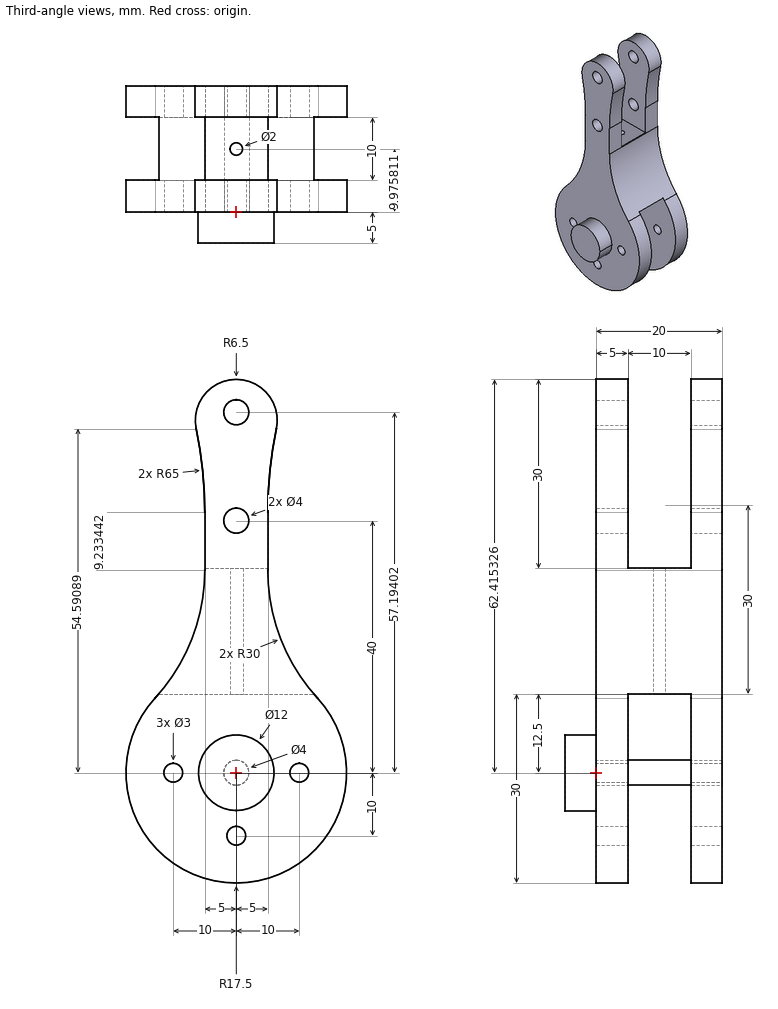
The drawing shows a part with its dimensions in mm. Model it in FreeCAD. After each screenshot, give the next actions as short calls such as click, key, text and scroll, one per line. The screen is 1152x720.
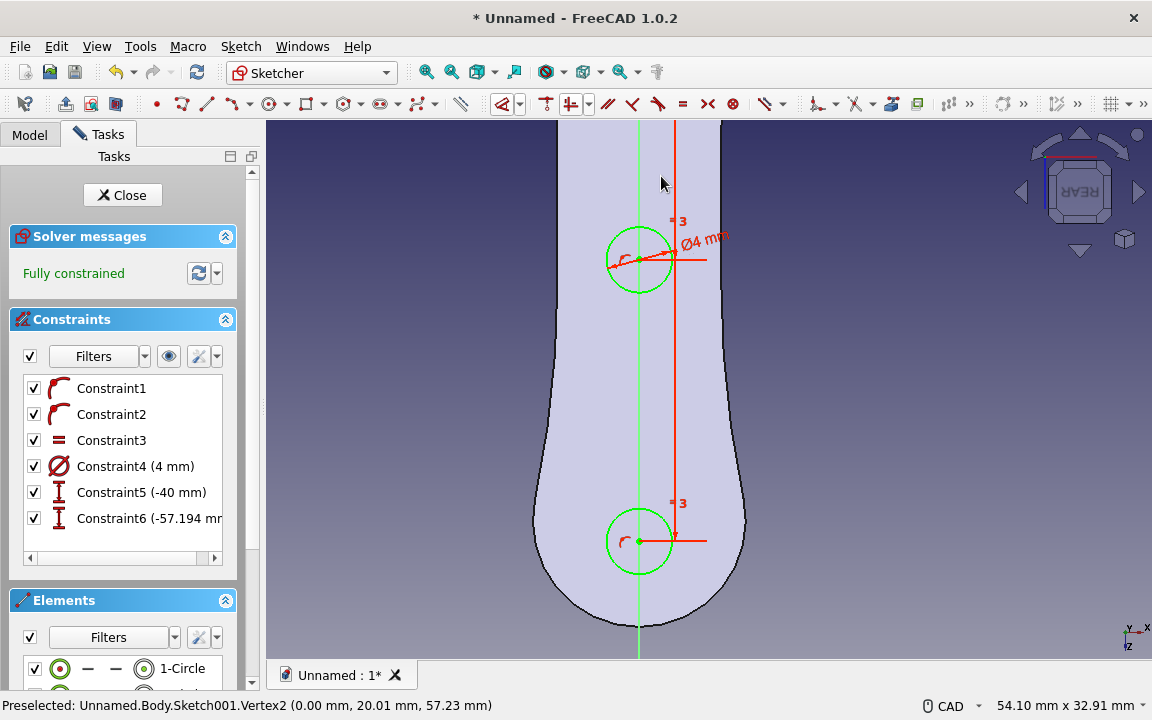
click(123, 195)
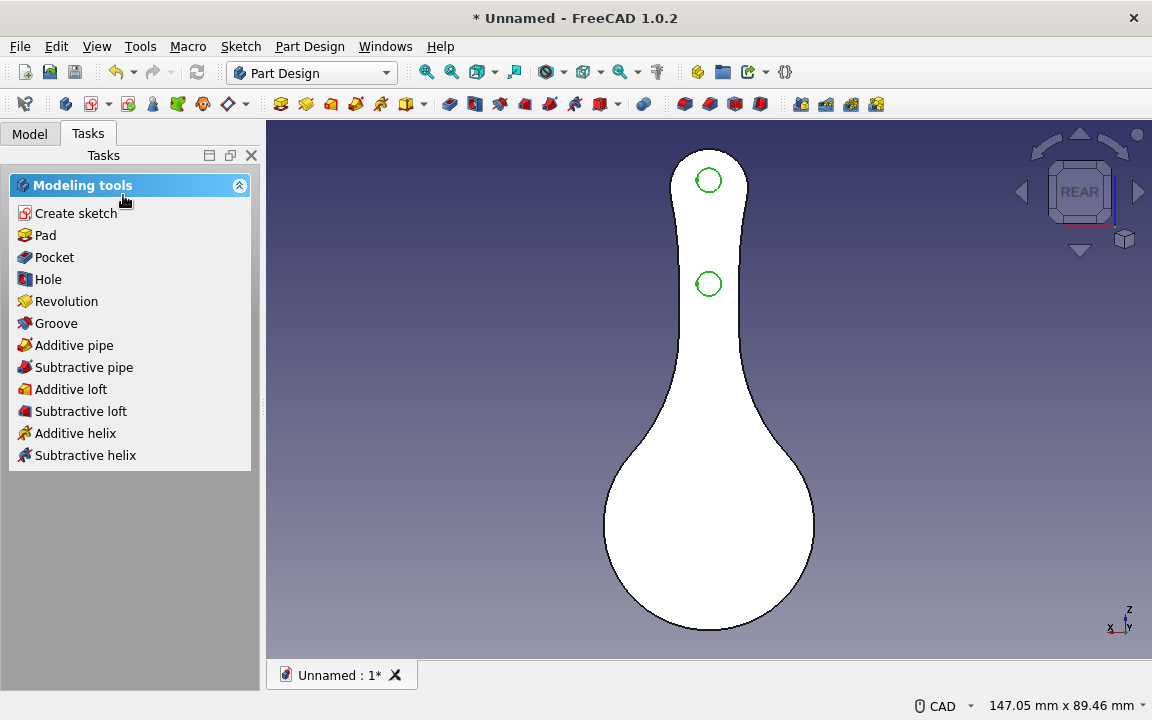
click(450, 104)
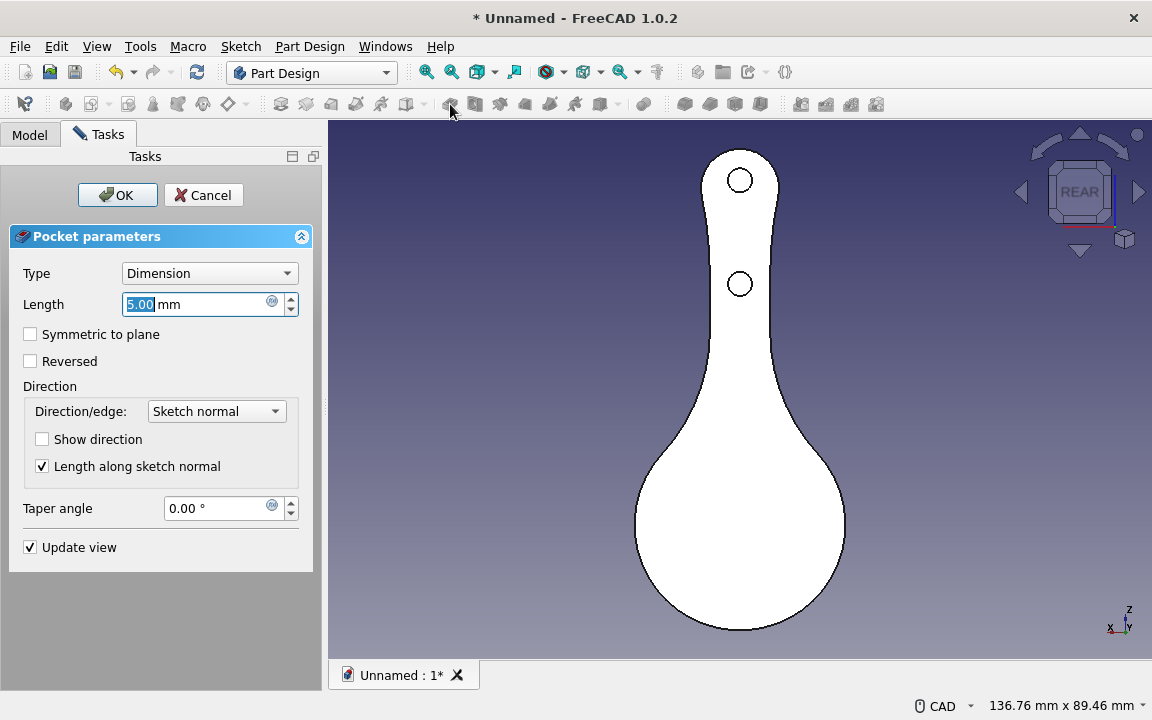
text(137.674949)
key(Tab)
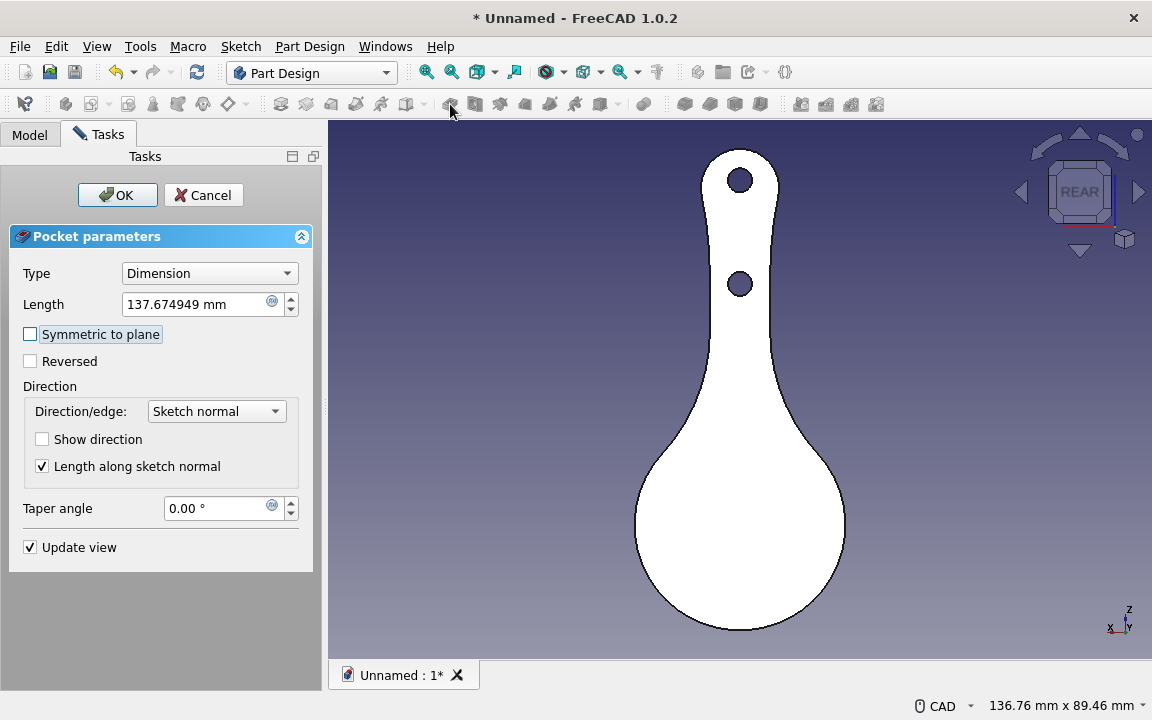
click(31, 334)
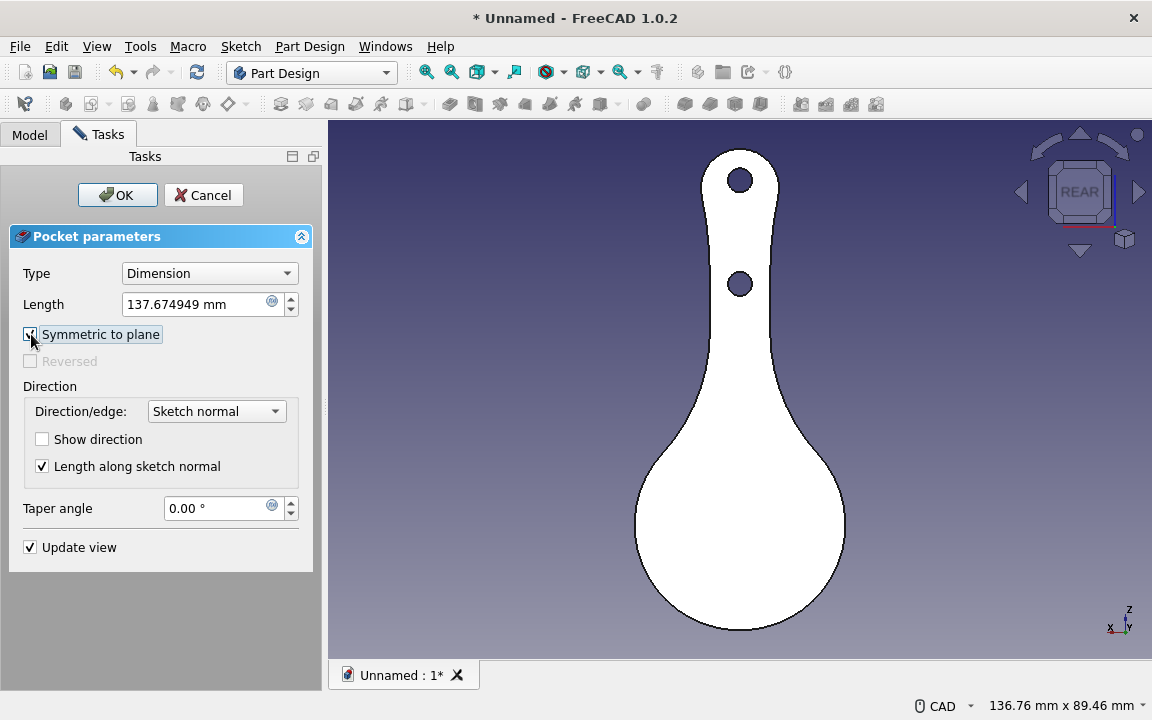
click(118, 195)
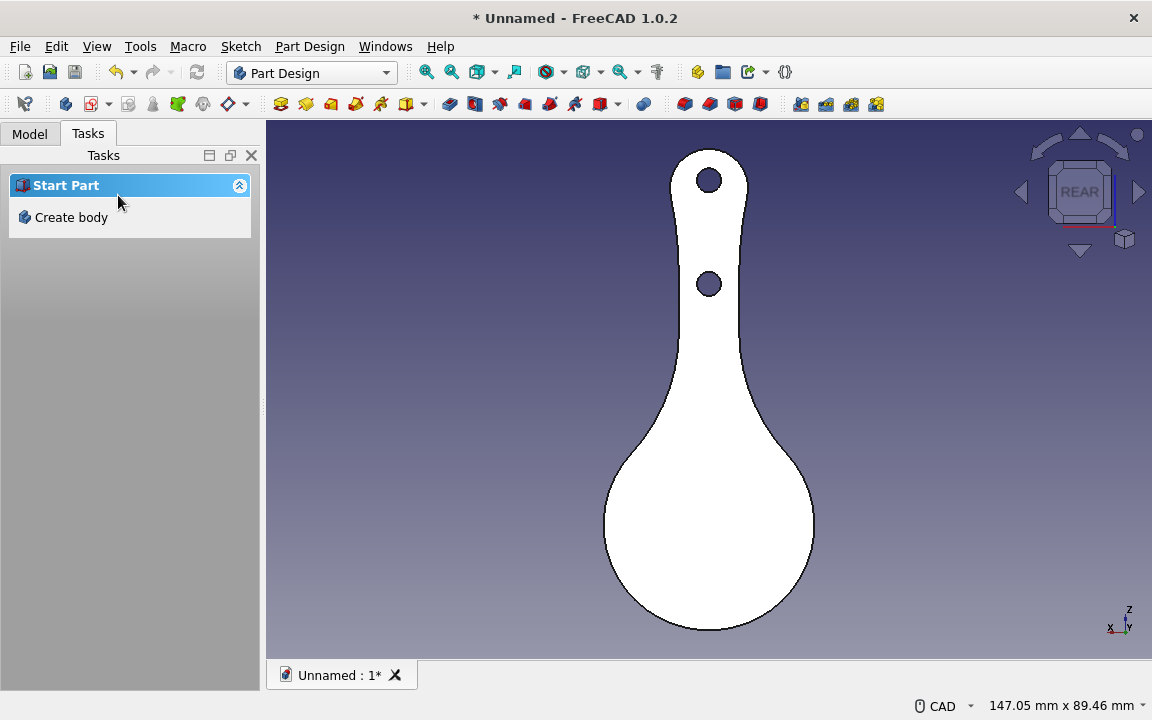
click(709, 526)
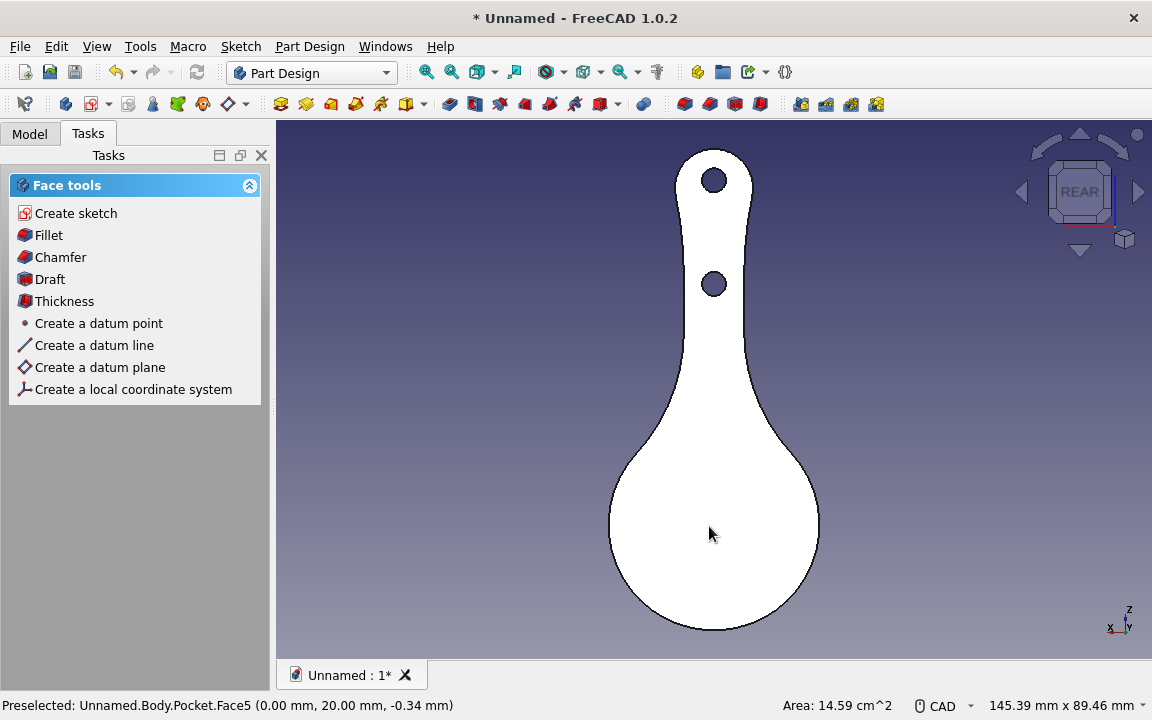
click(90, 104)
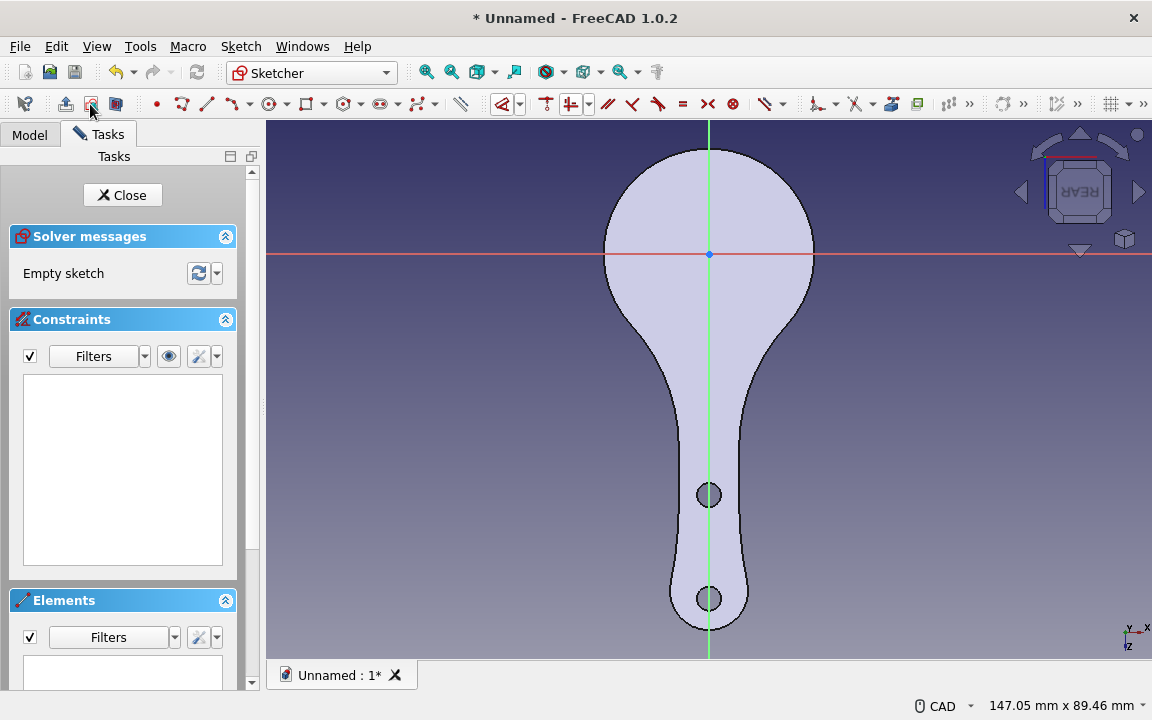
scroll(714, 243, up, 13)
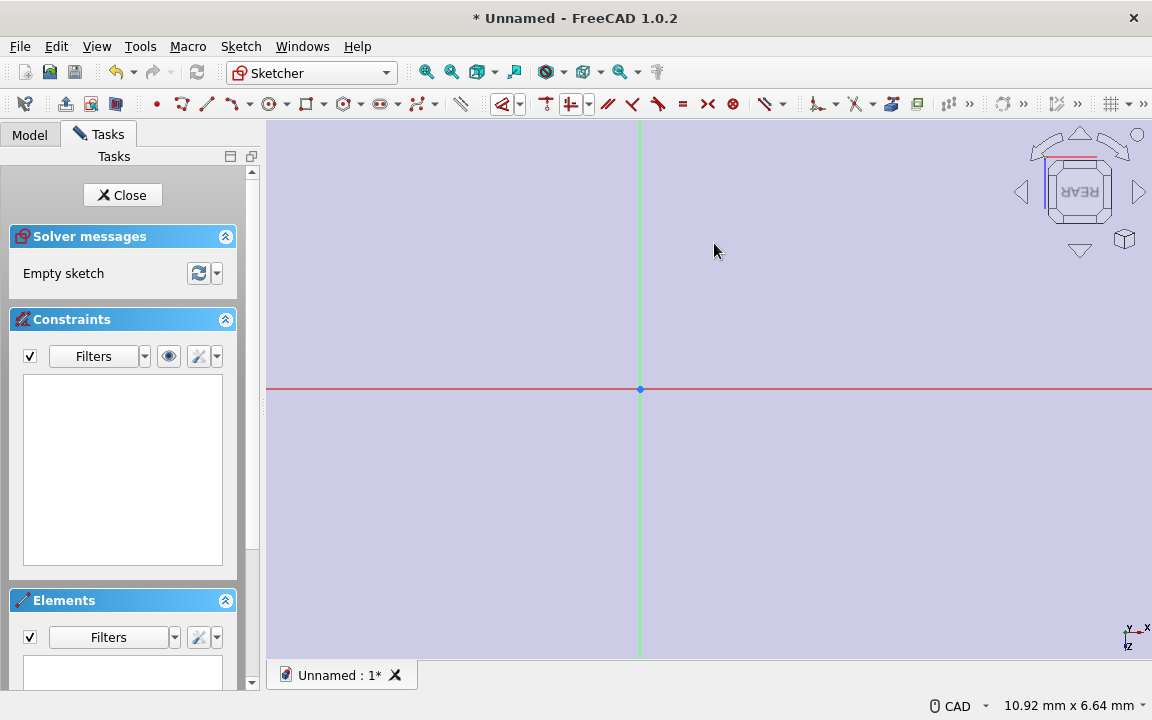
click(268, 104)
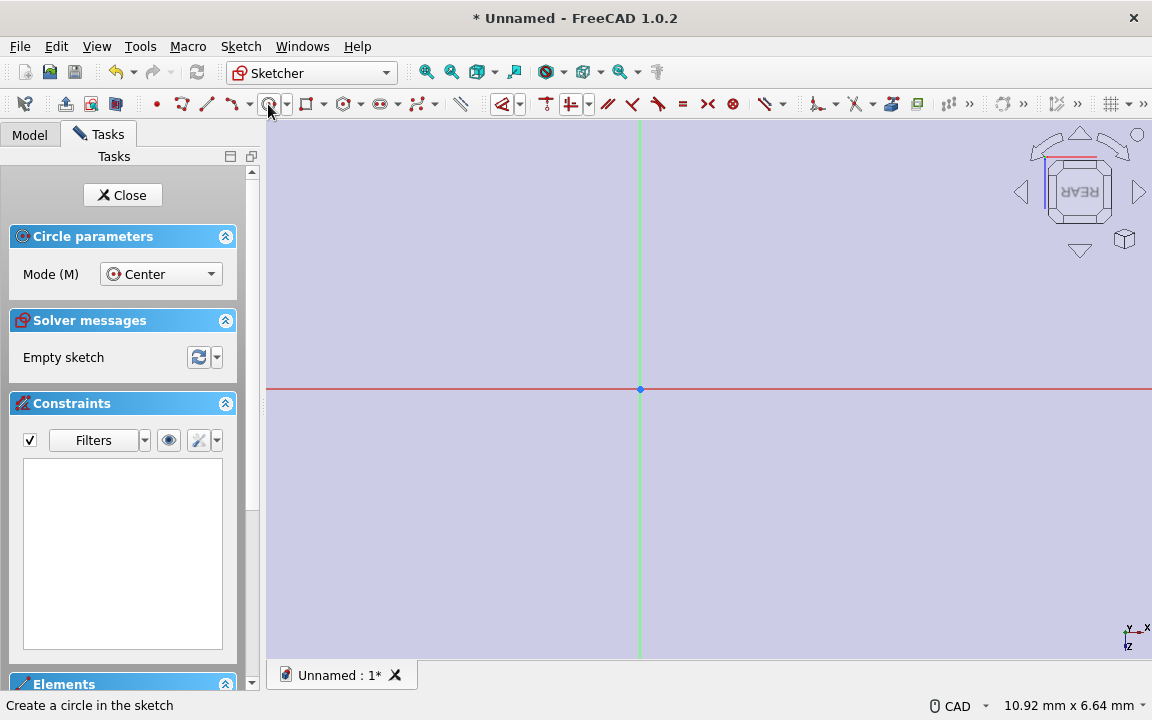
click(640, 389)
click(755, 274)
key(Escape)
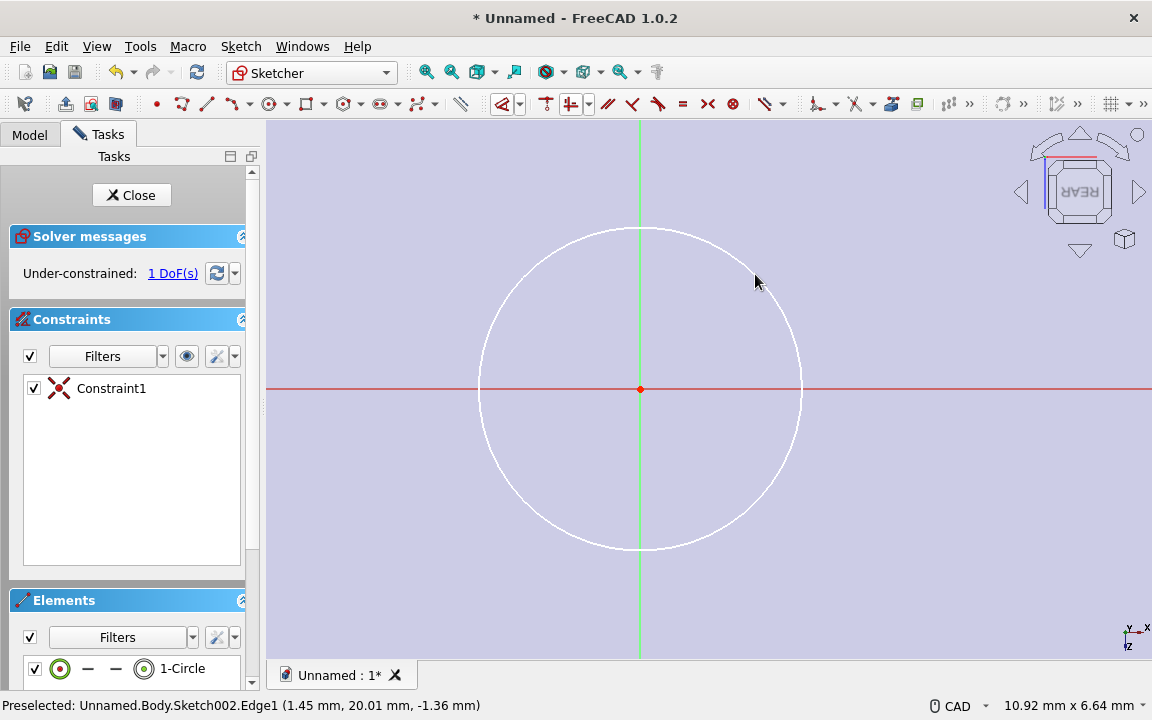
click(754, 274)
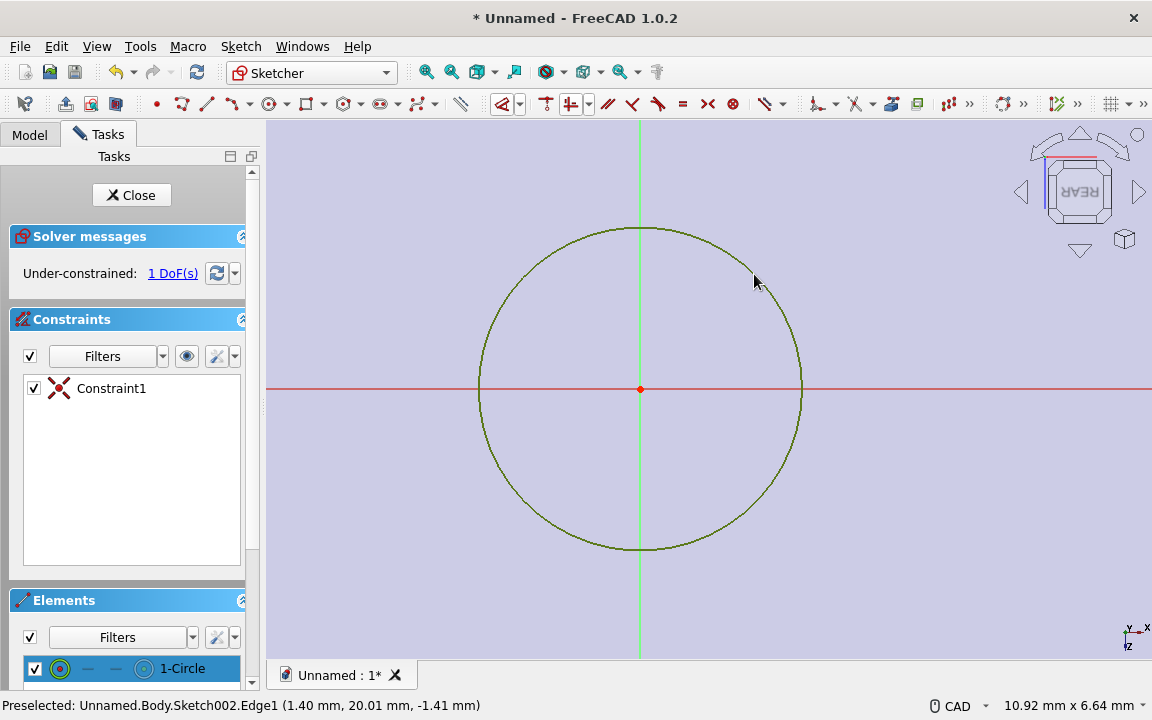
click(520, 104)